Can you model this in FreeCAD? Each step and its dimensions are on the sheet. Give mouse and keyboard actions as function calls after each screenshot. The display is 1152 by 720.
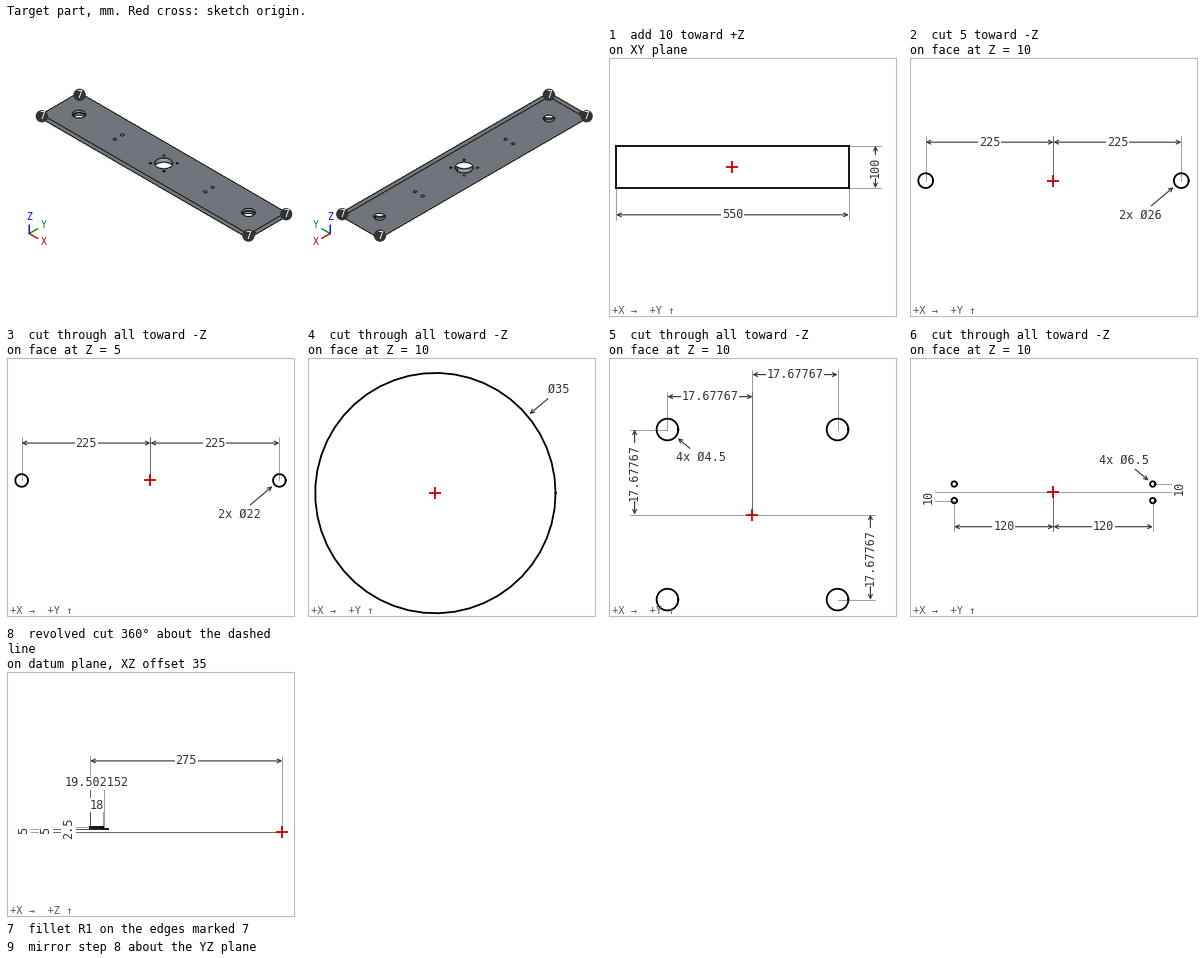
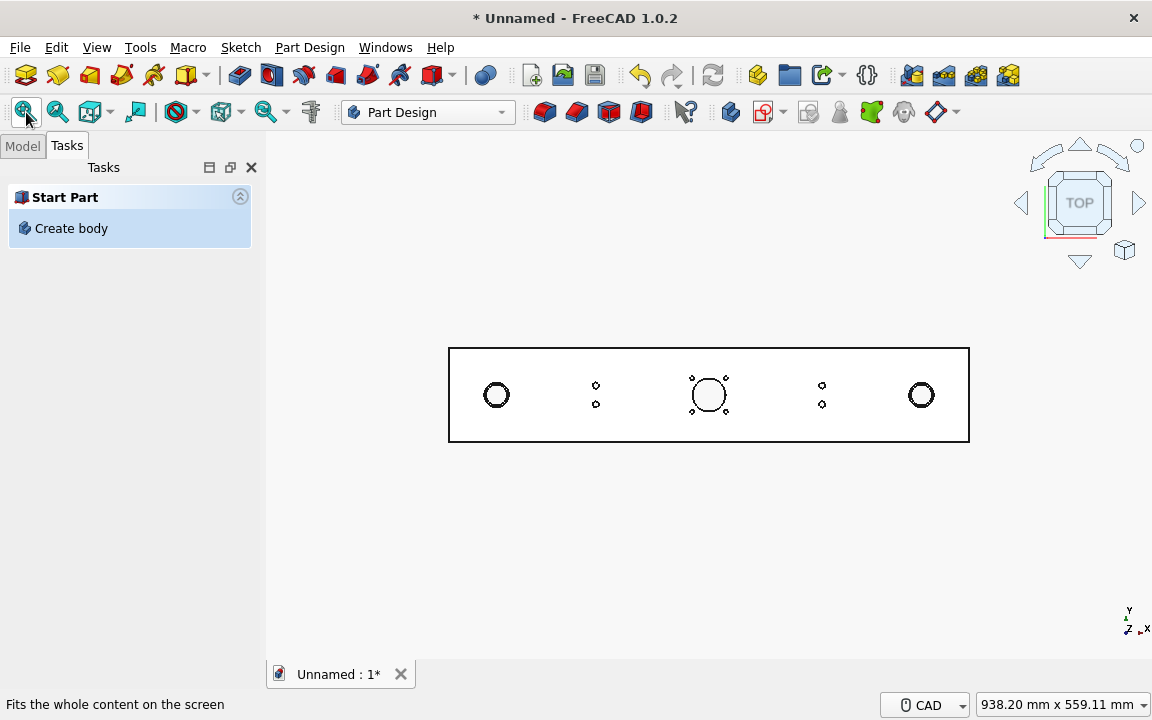
key(0)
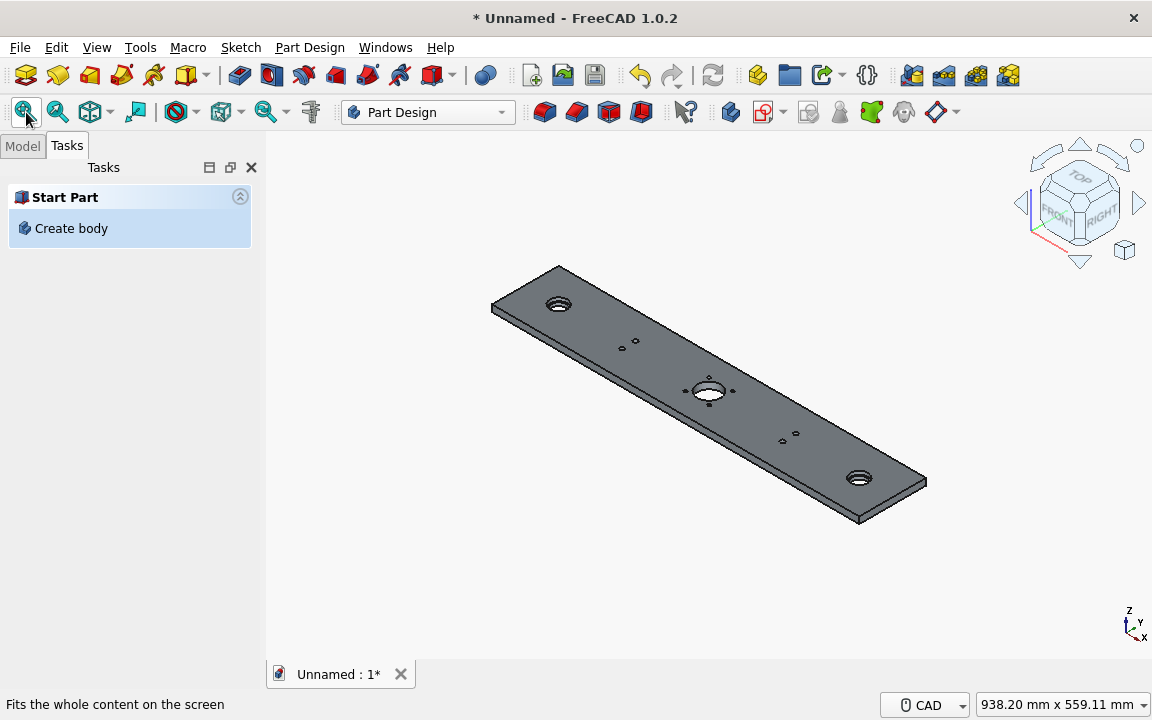
click(859, 522)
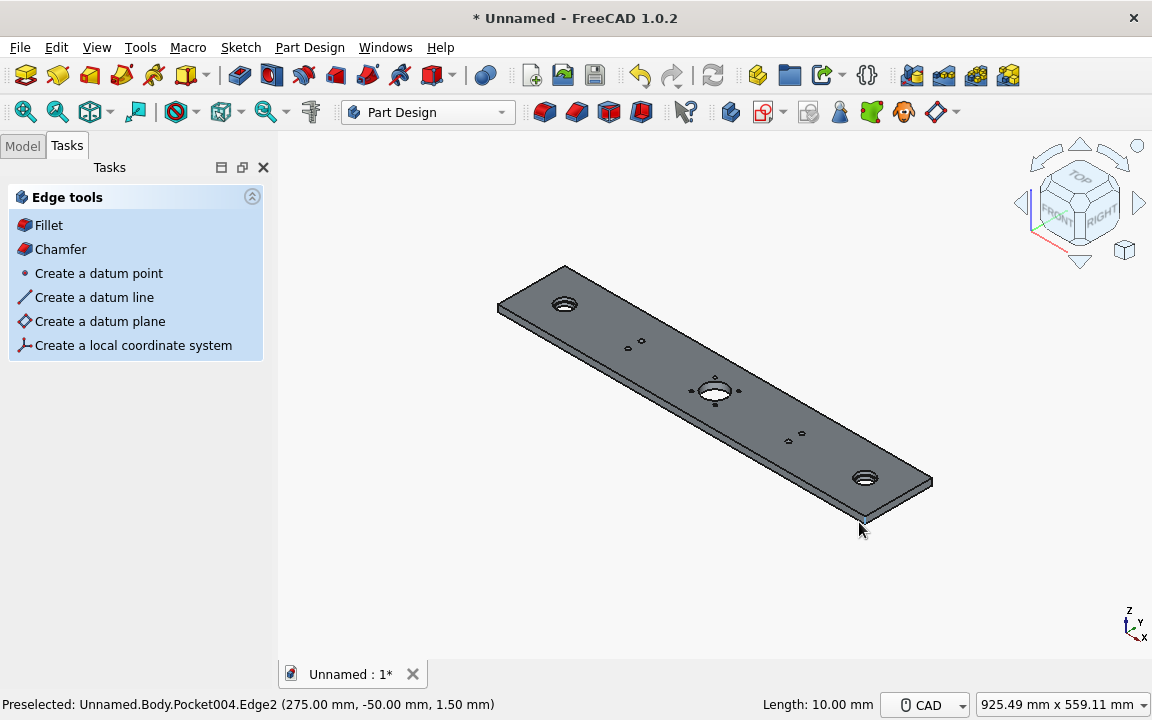
scroll(565, 269, up, 8)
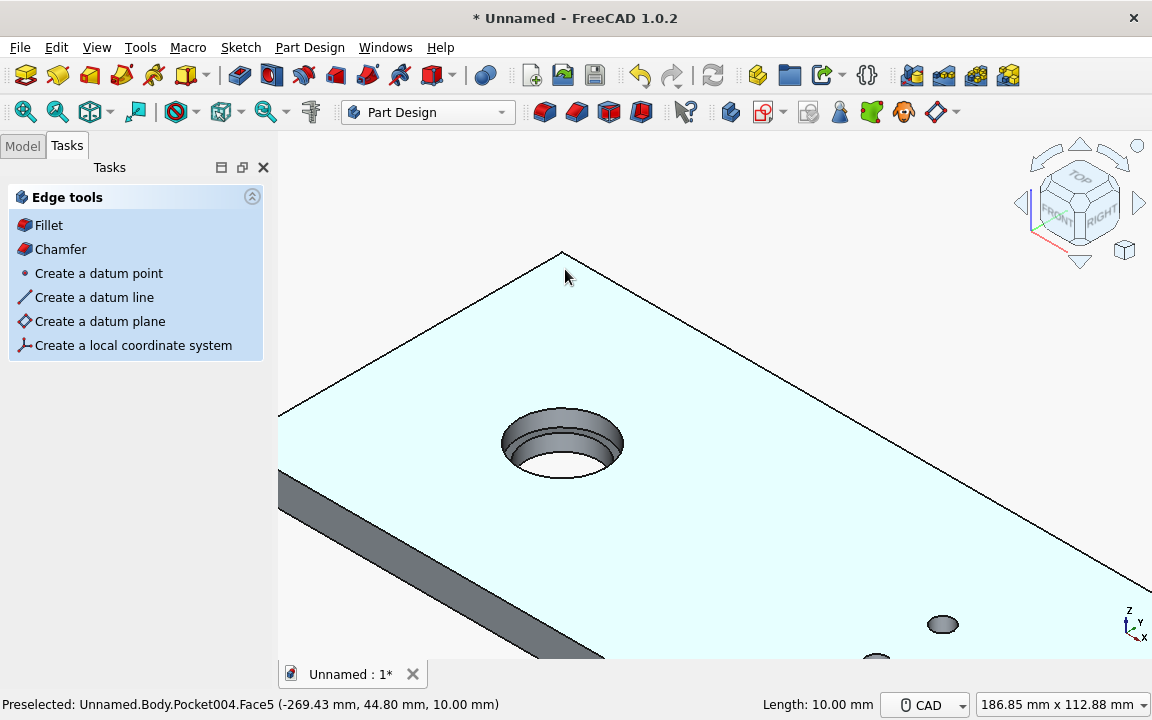
click(26, 112)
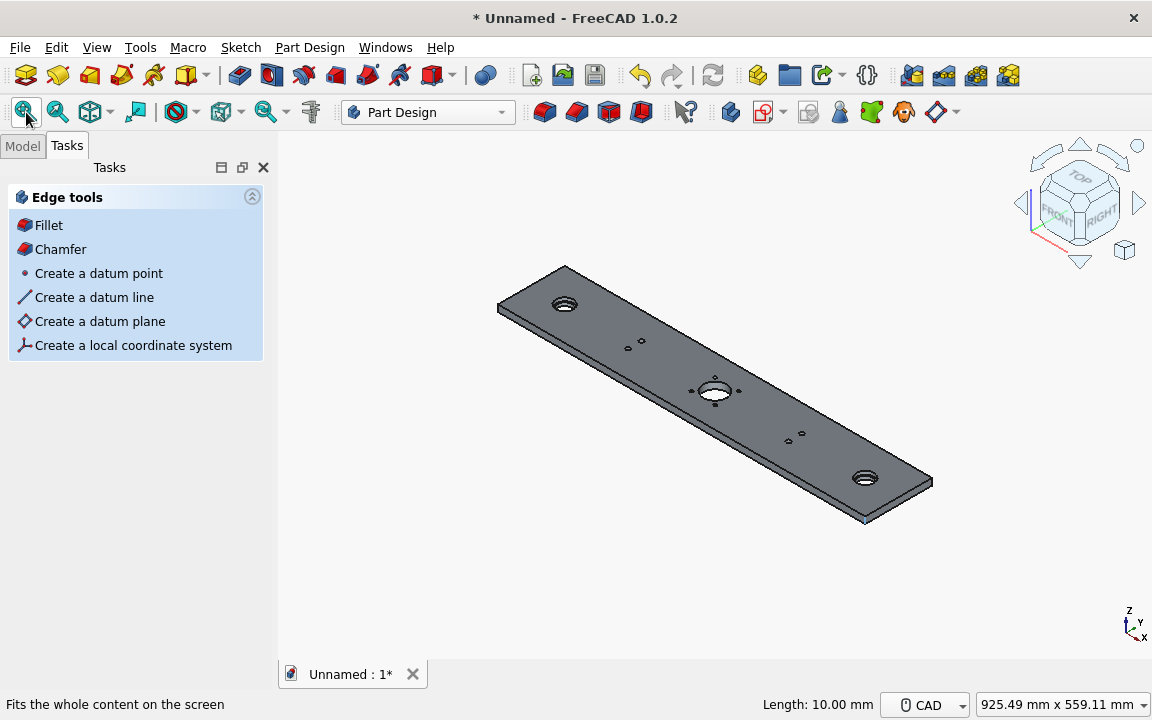
key(2)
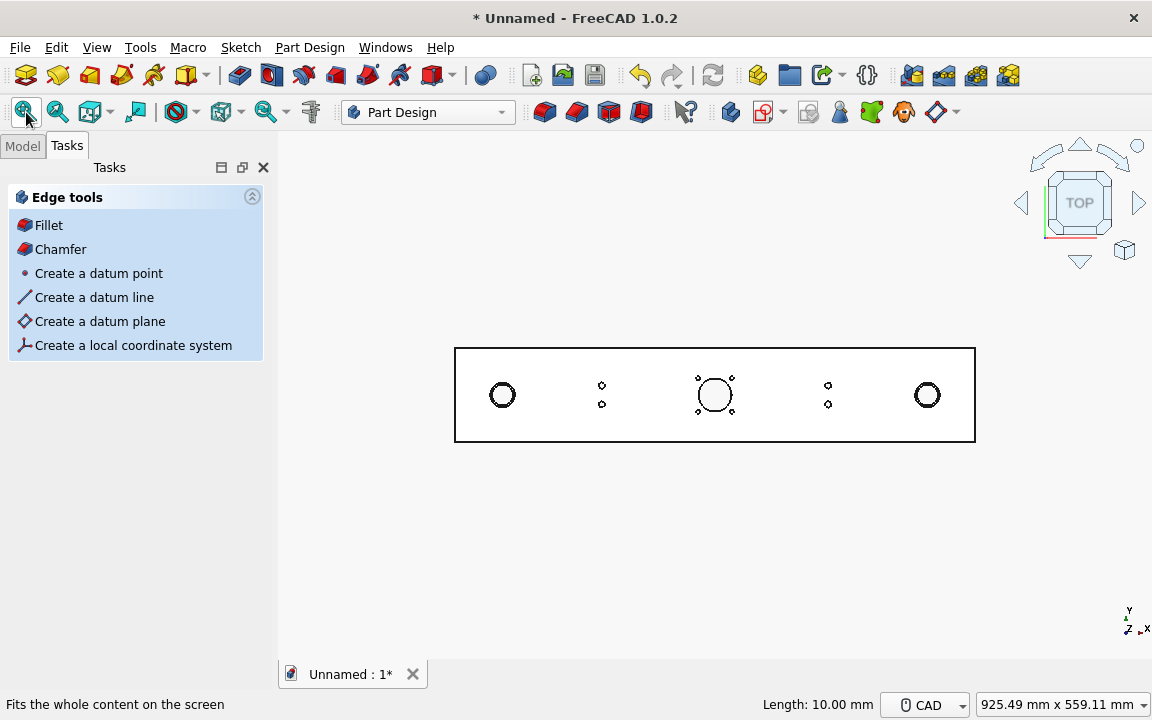
scroll(455, 347, up, 8)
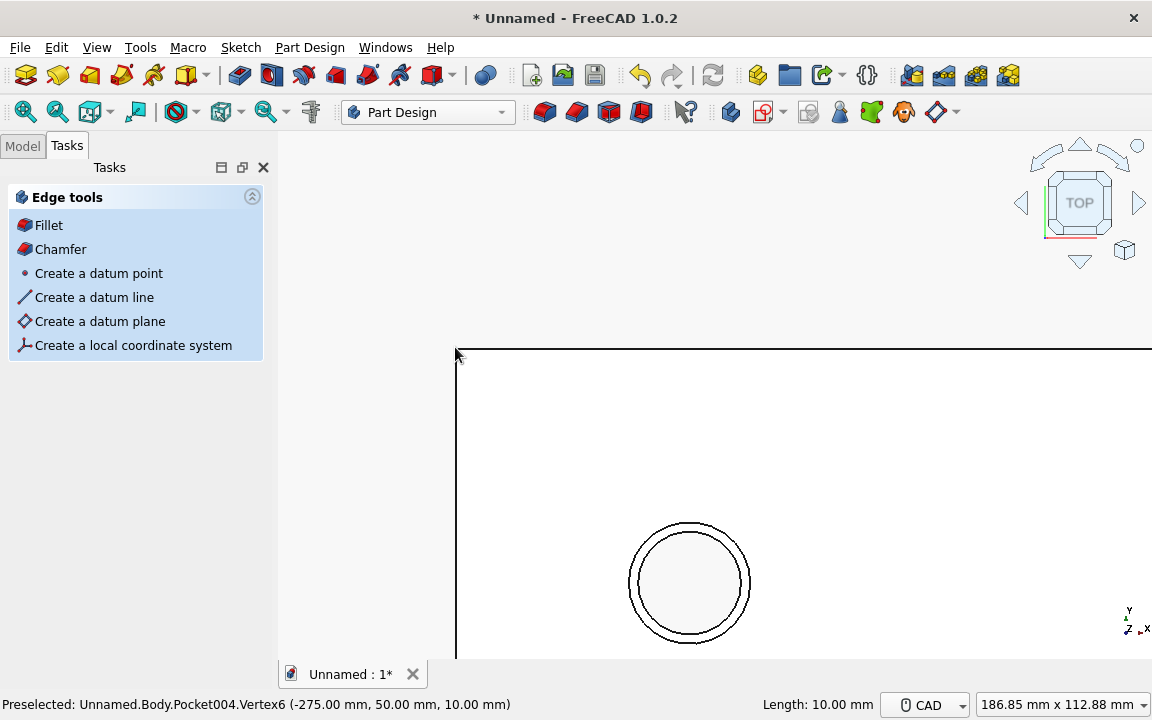
click(26, 112)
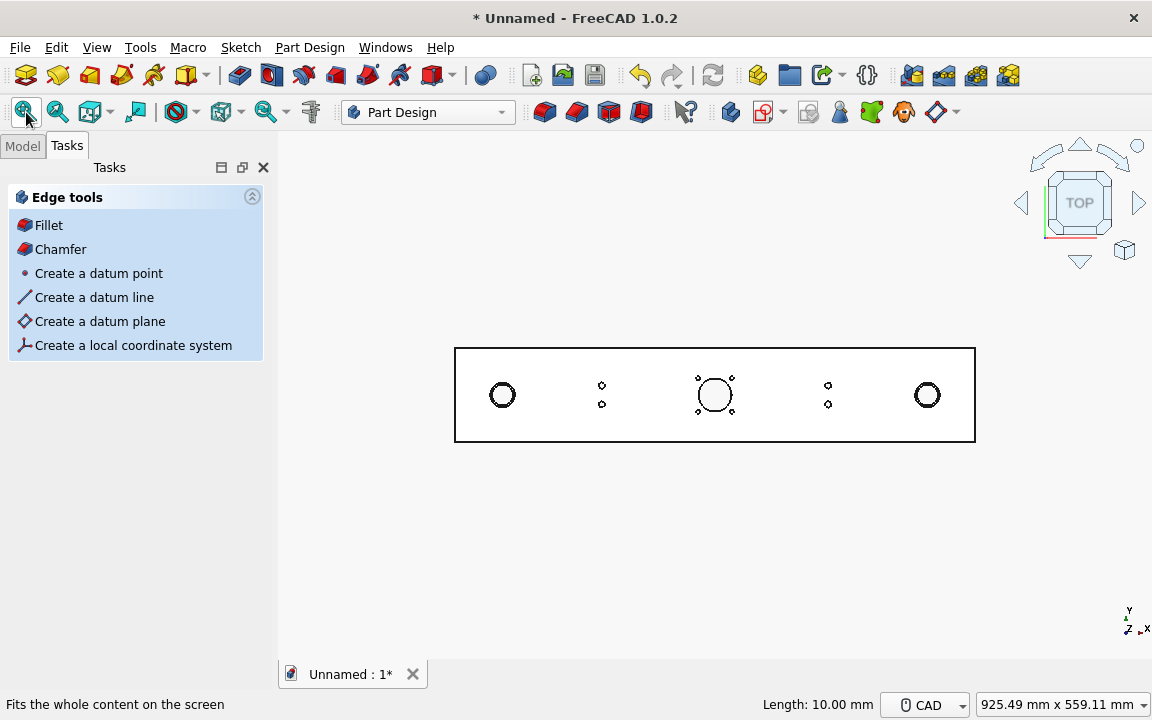
key(1)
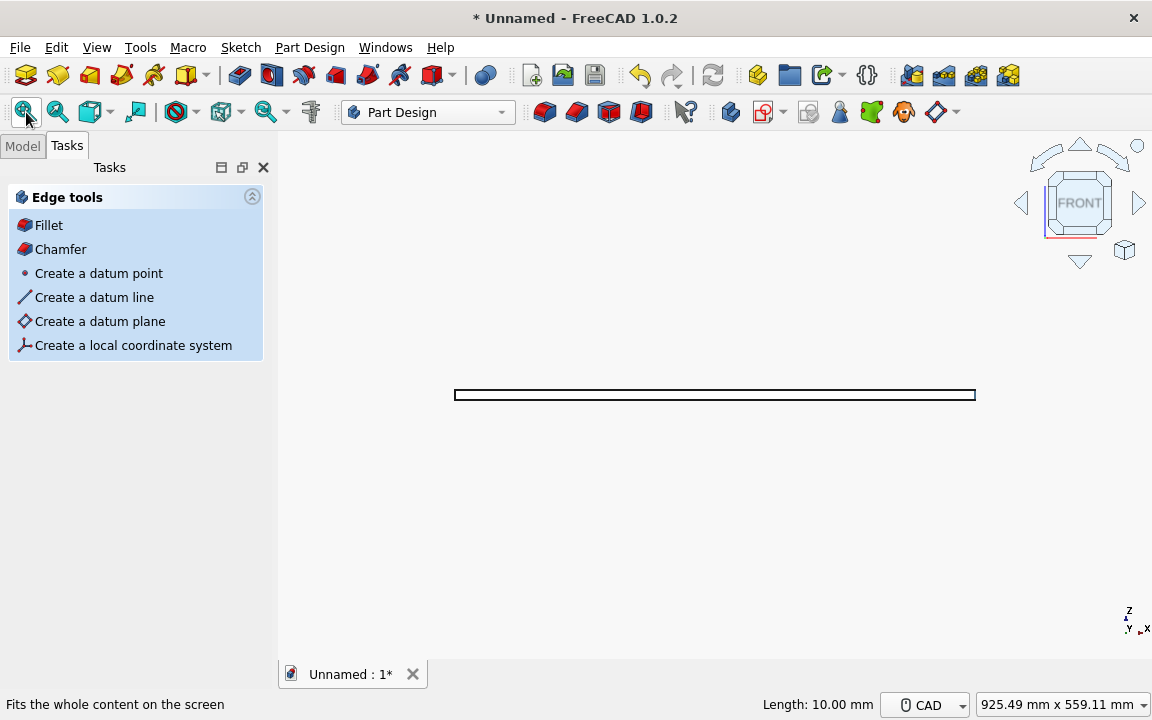
scroll(455, 394, up, 8)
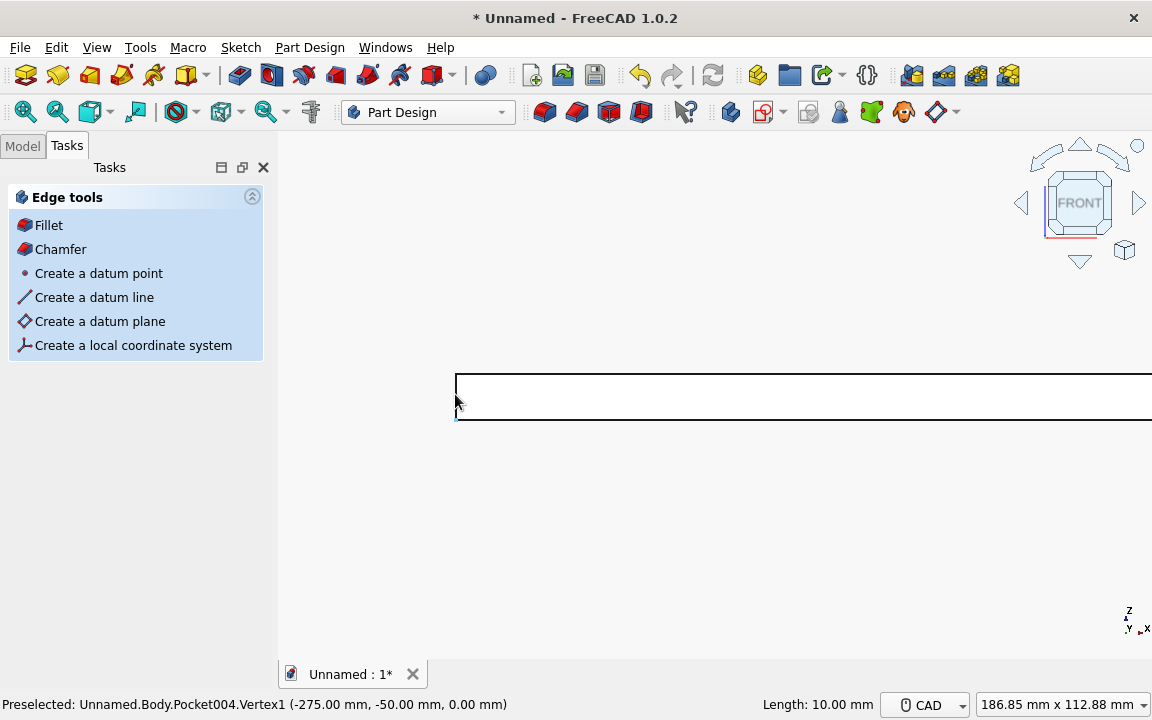
click(456, 396, ctrl)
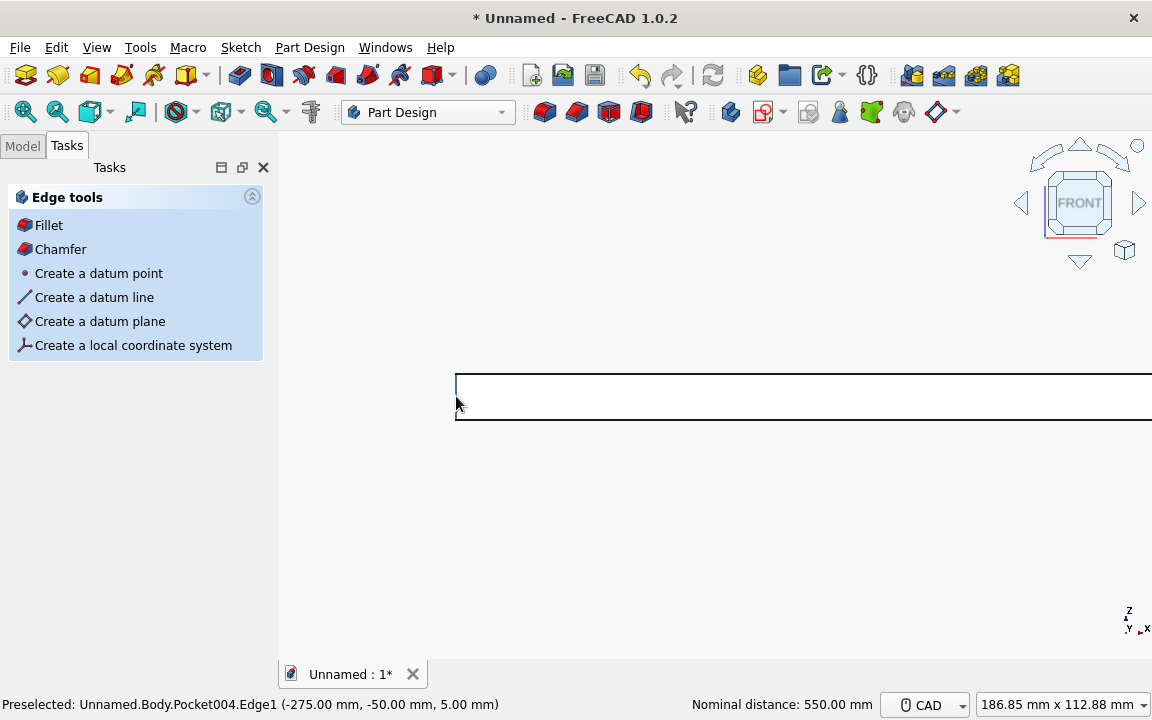
click(26, 112)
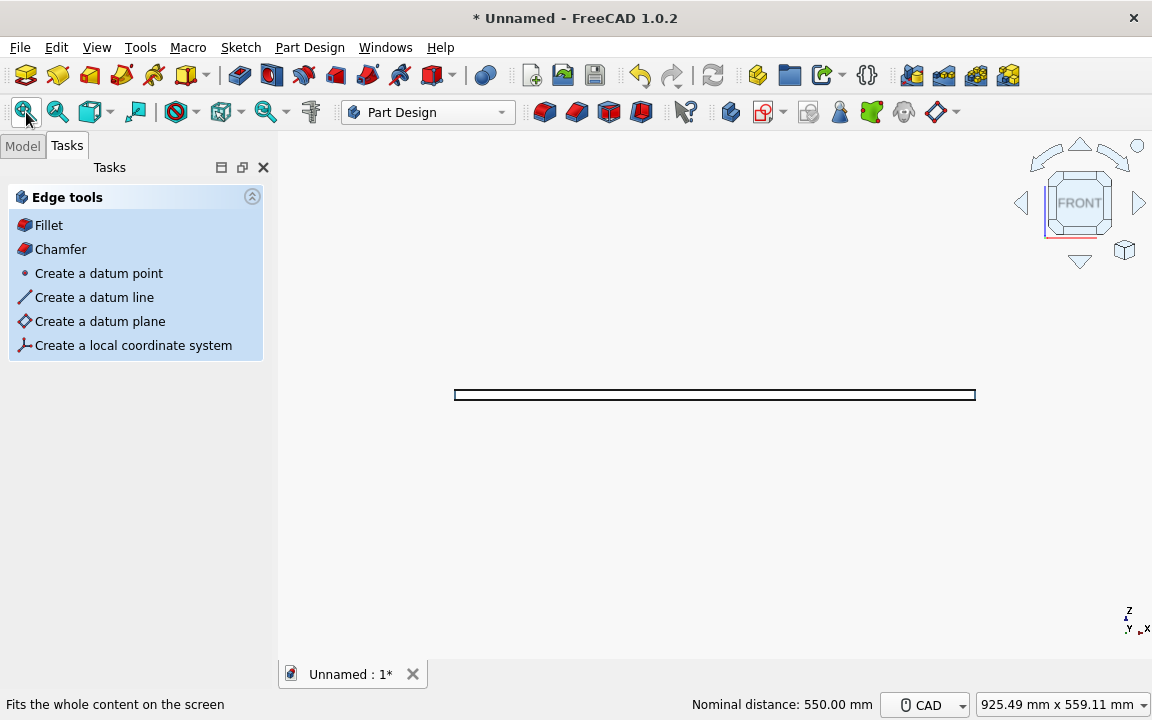
key(3)